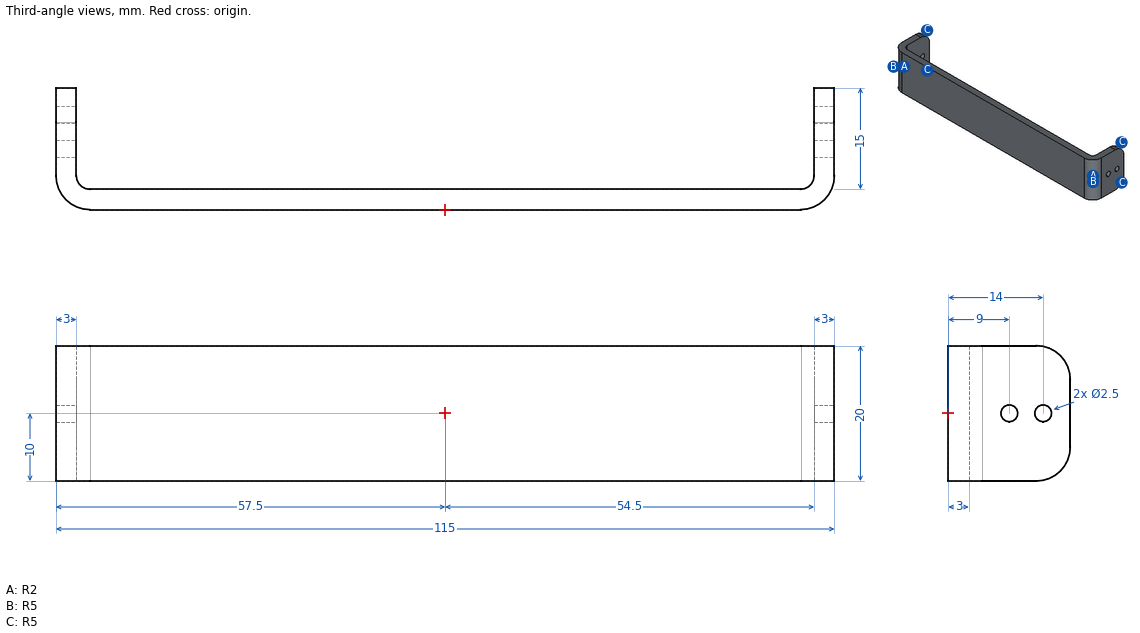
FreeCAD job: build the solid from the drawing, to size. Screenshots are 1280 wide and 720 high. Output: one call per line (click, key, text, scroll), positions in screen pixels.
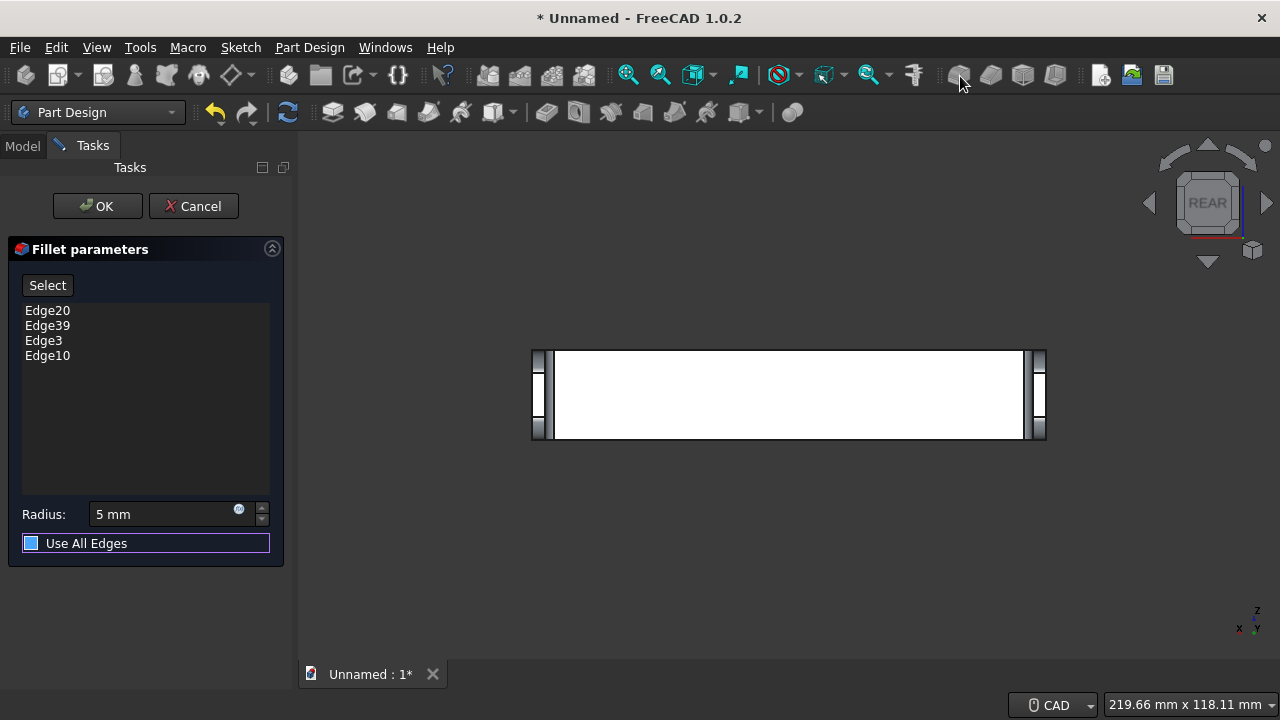
click(98, 206)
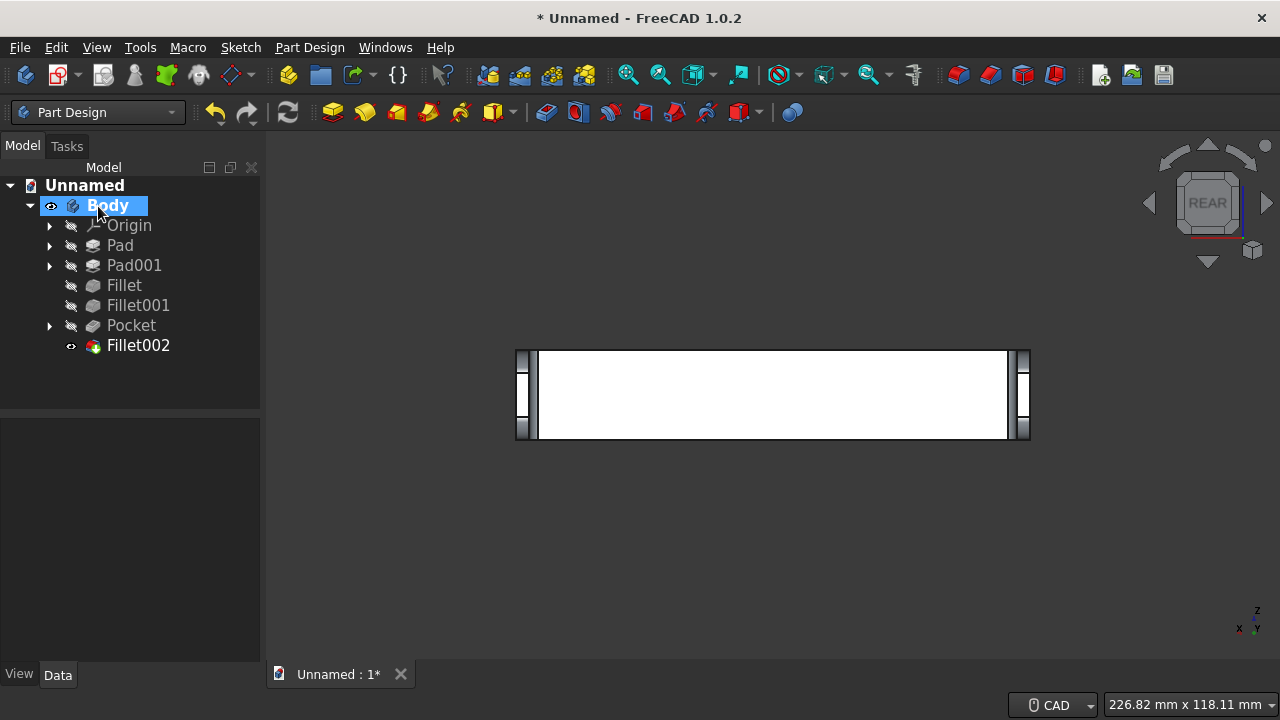
key(0)